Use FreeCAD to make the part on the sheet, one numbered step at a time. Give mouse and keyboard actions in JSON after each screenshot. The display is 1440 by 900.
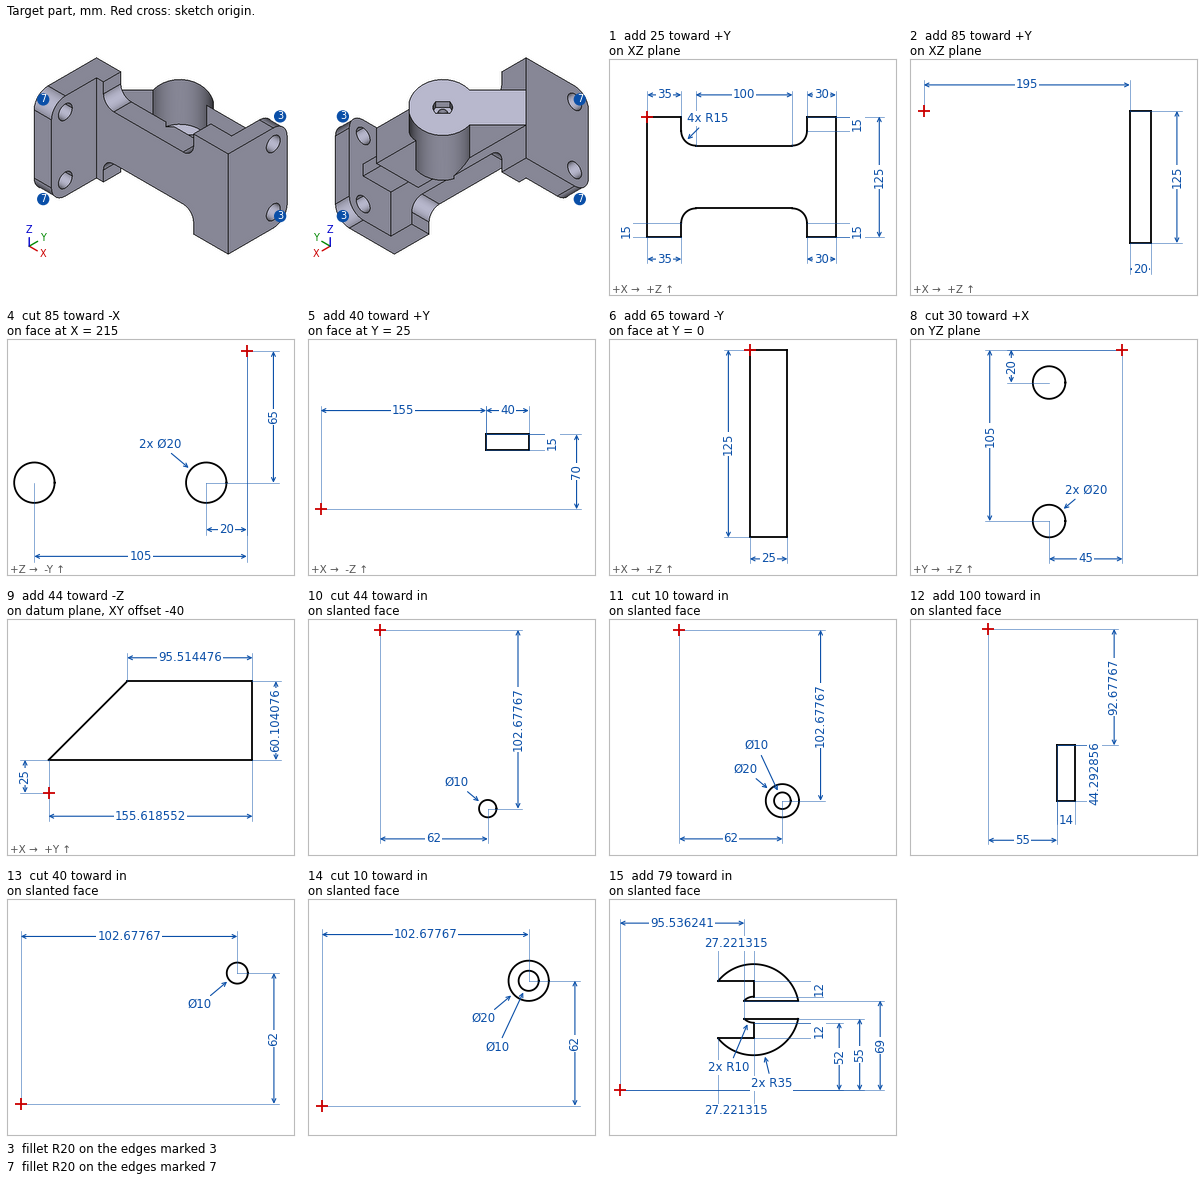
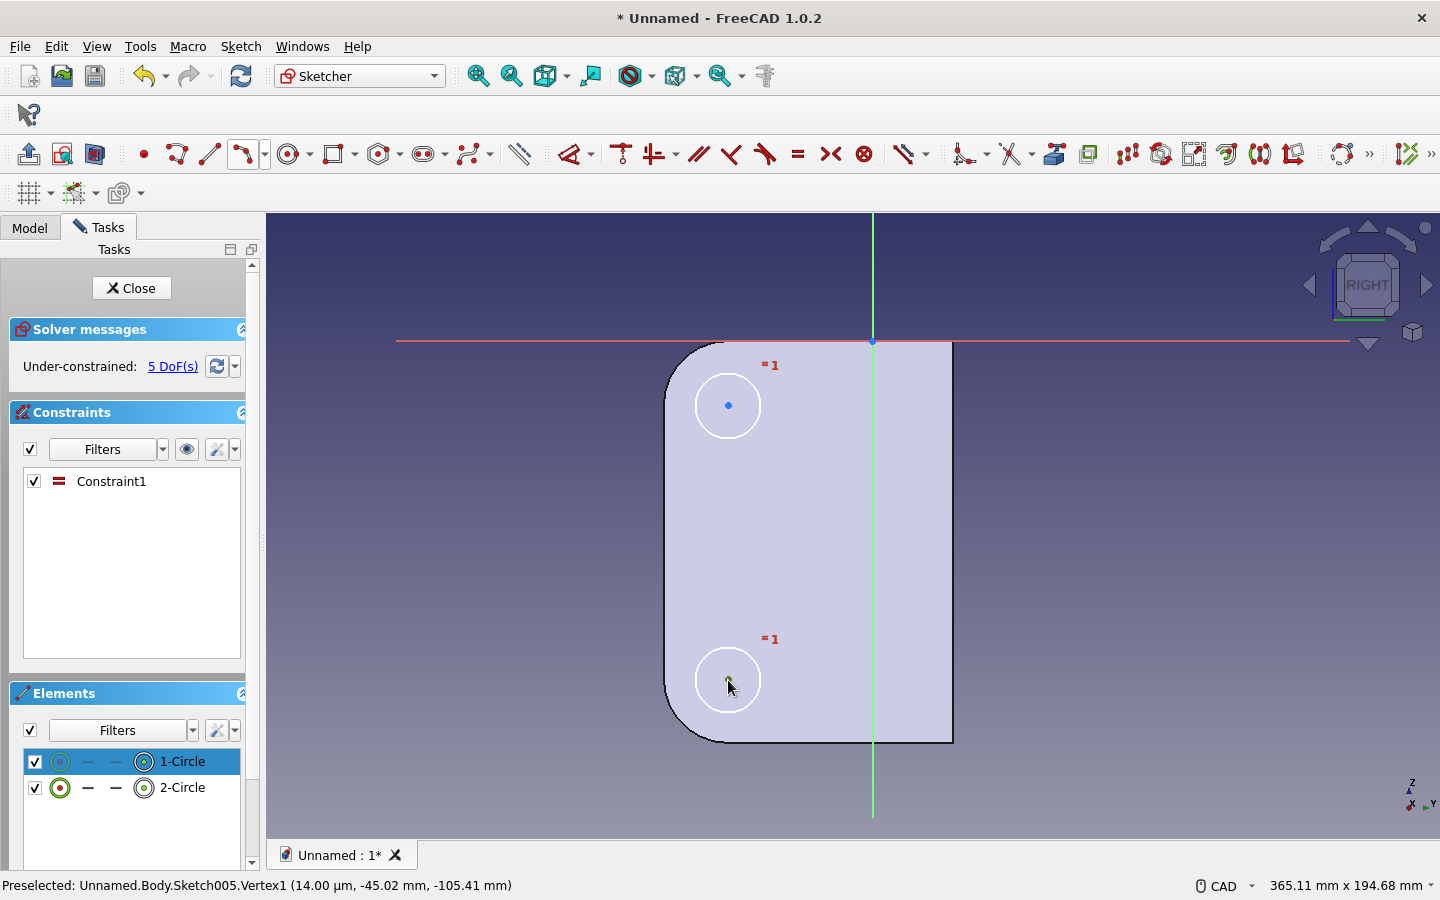
{"action": "left_click", "coordinate": [728, 406]}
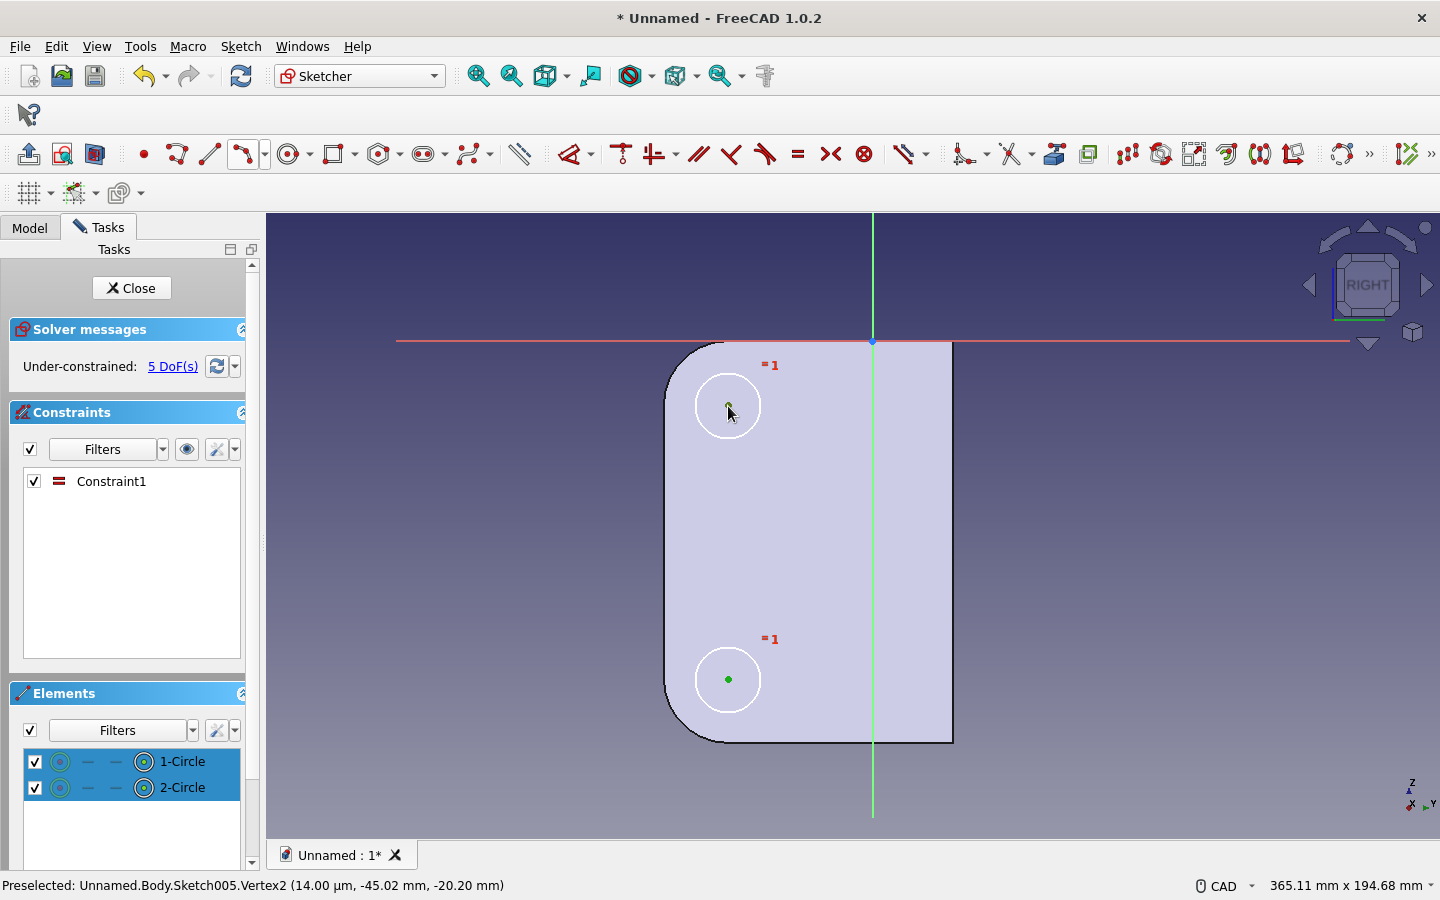
{"action": "left_click", "coordinate": [676, 154]}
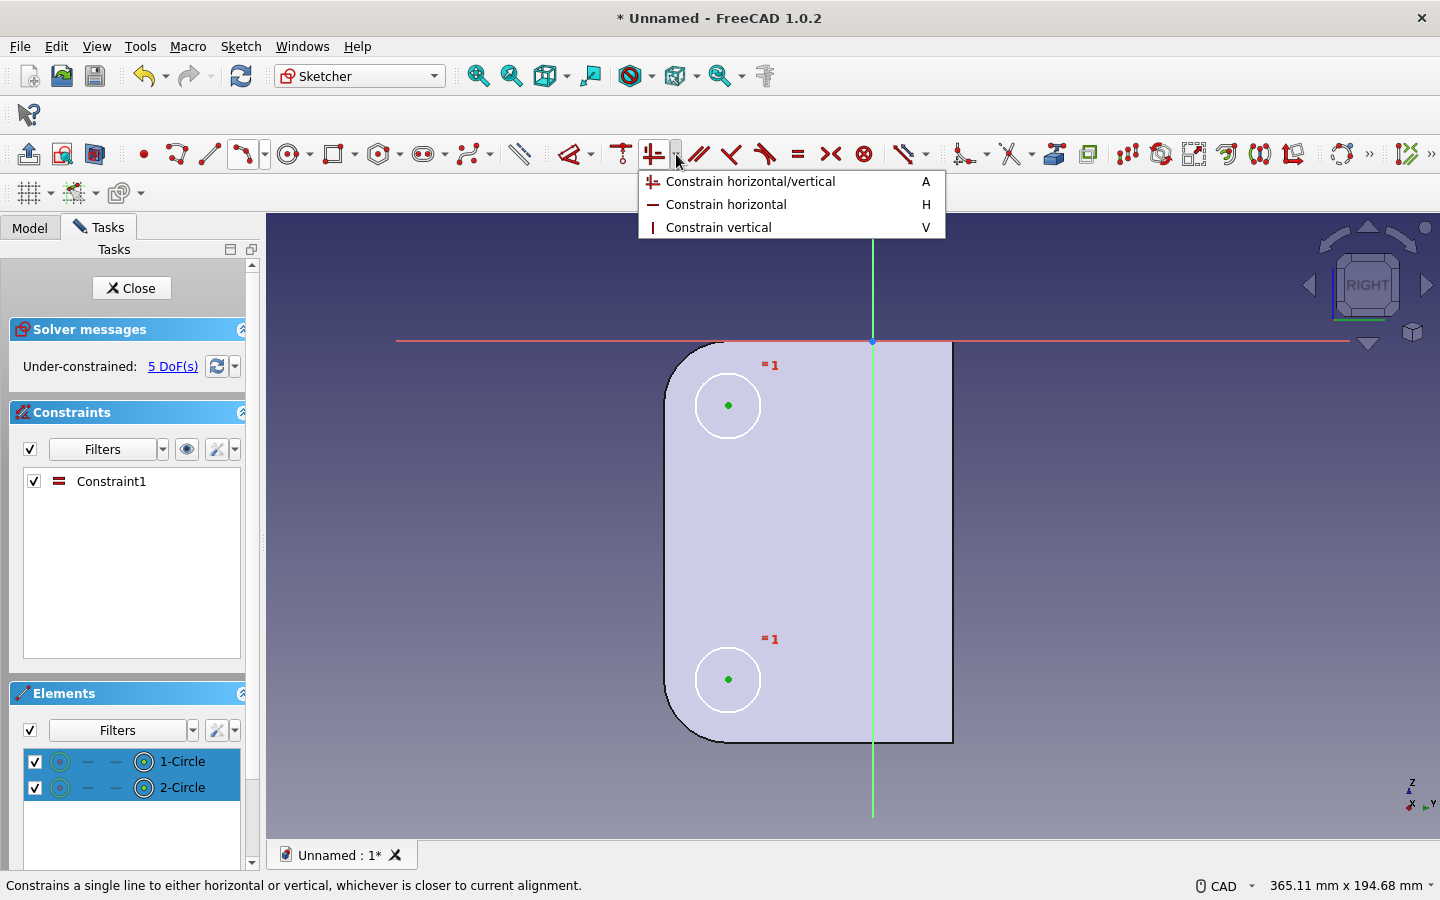
{"action": "left_click", "coordinate": [792, 228]}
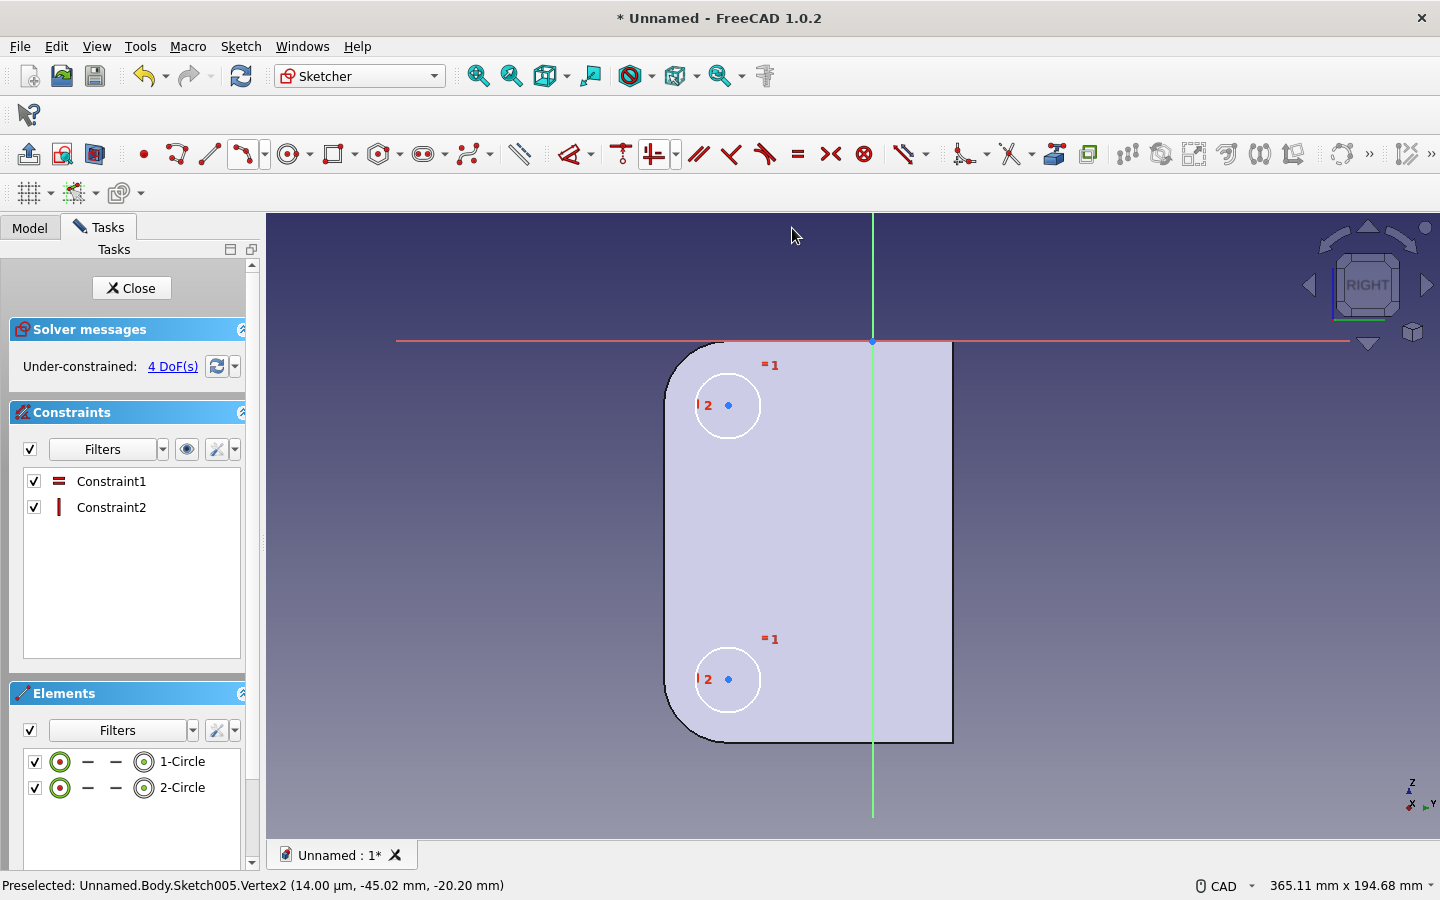
{"action": "left_click", "coordinate": [568, 154]}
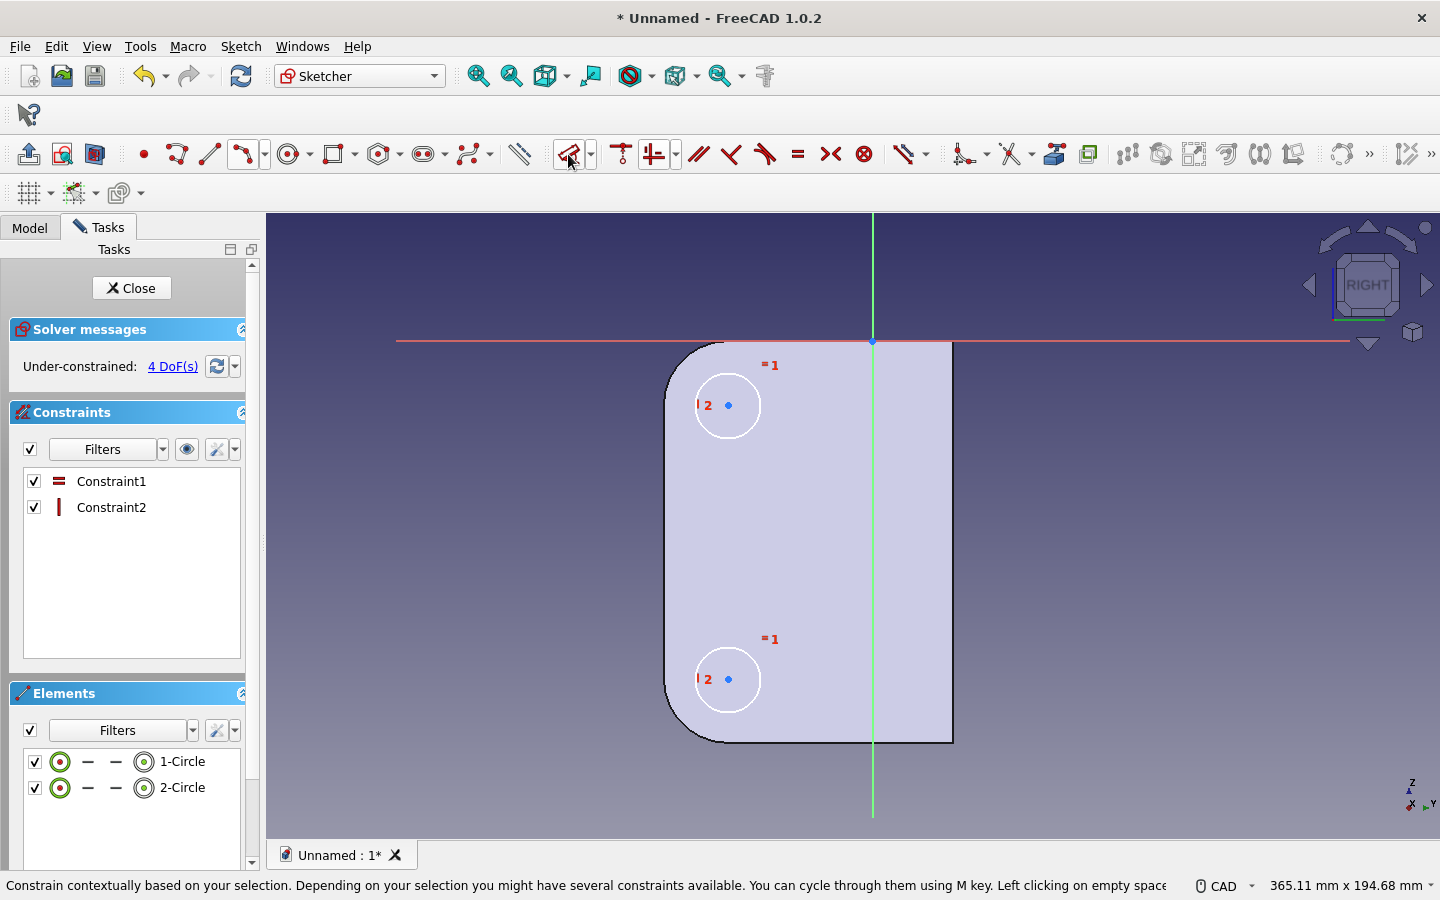
{"action": "left_click", "coordinate": [751, 657]}
{"action": "left_click", "coordinate": [774, 634]}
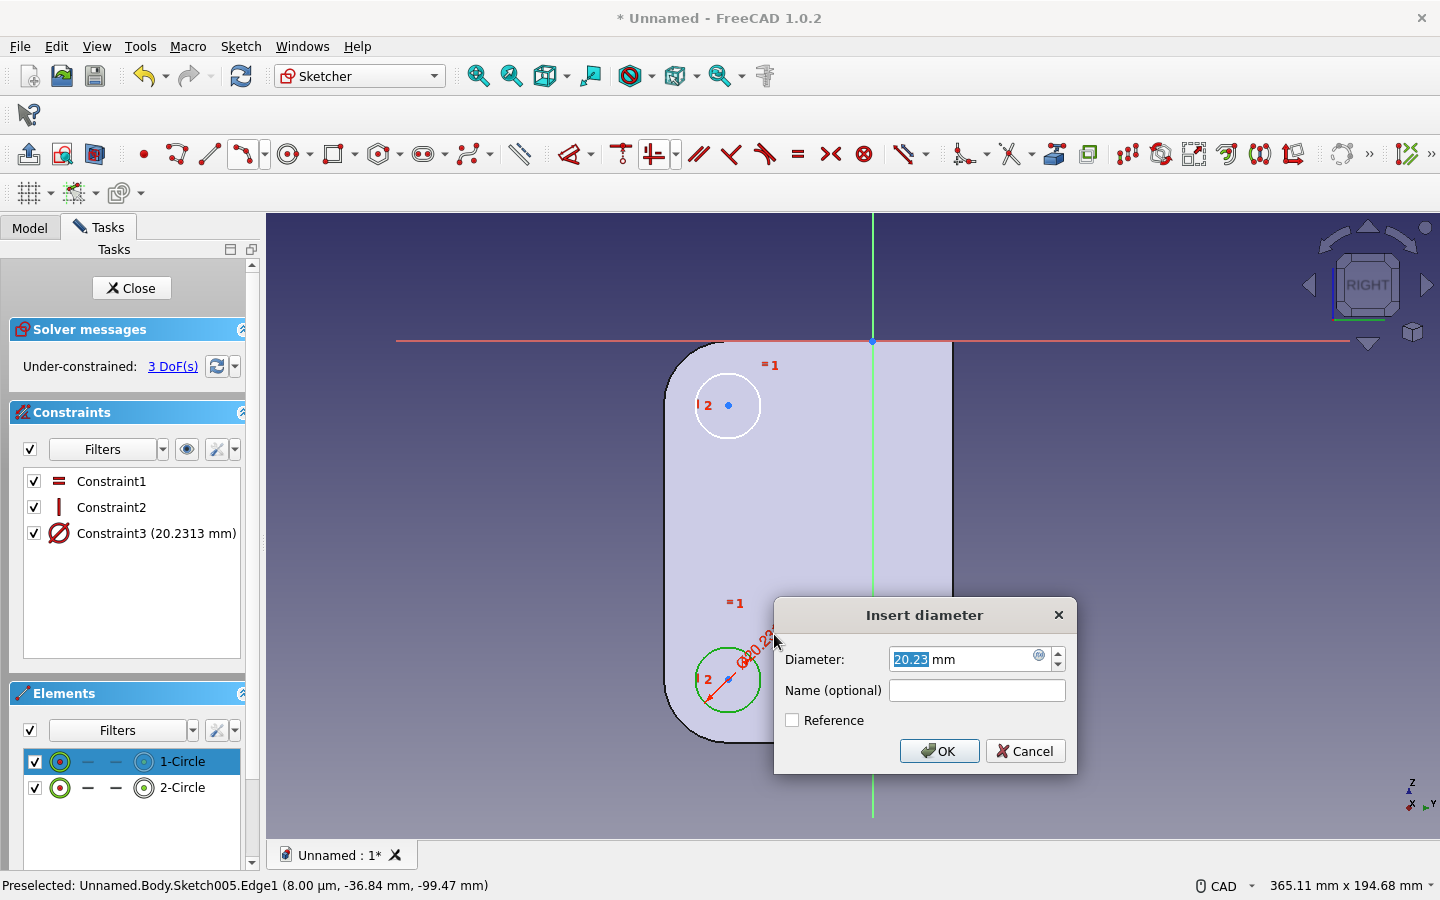
{"action": "type", "text": "20"}
{"action": "key", "text": "Return"}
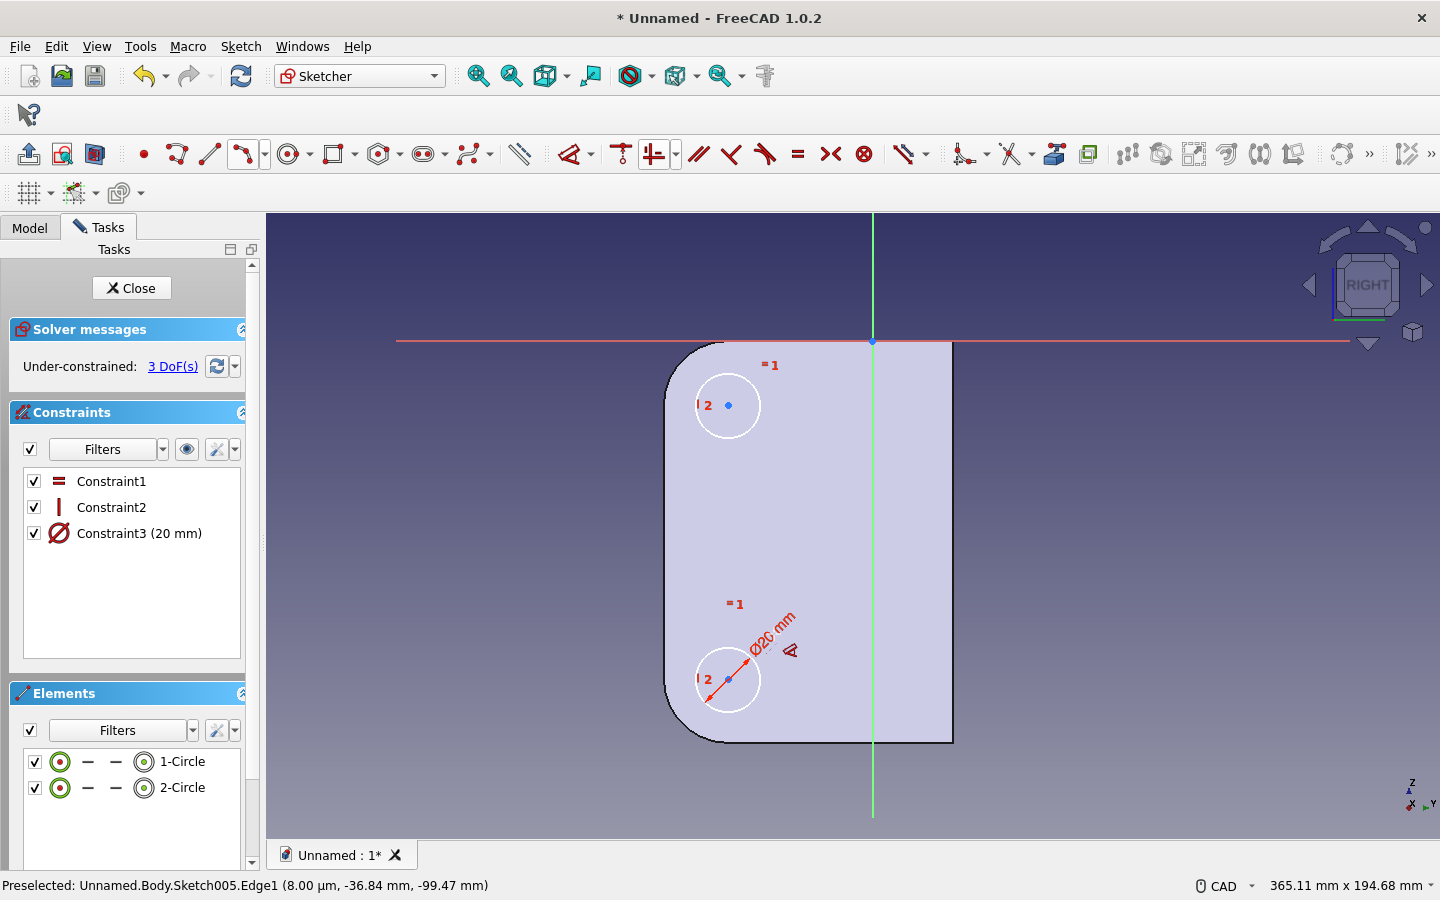
{"action": "left_click", "coordinate": [728, 680]}
{"action": "left_click", "coordinate": [800, 307]}